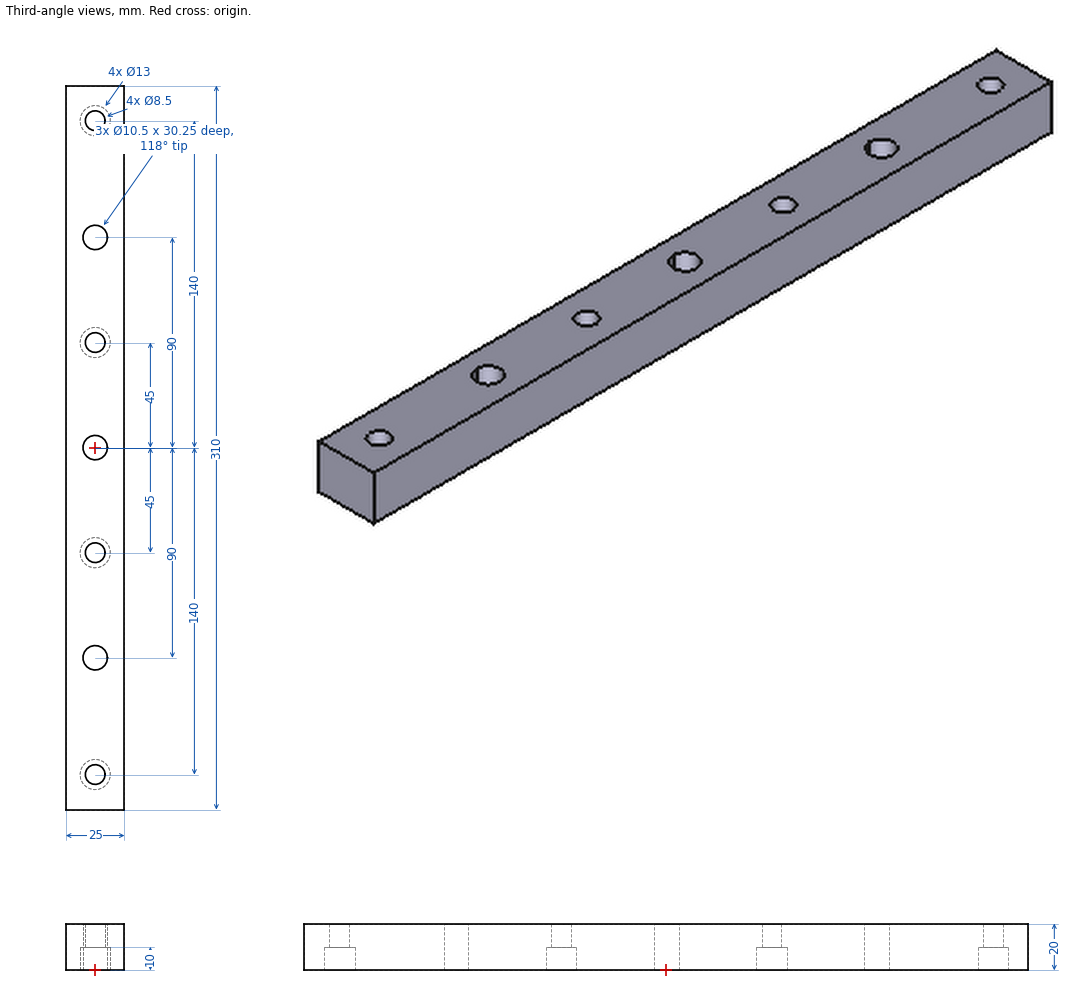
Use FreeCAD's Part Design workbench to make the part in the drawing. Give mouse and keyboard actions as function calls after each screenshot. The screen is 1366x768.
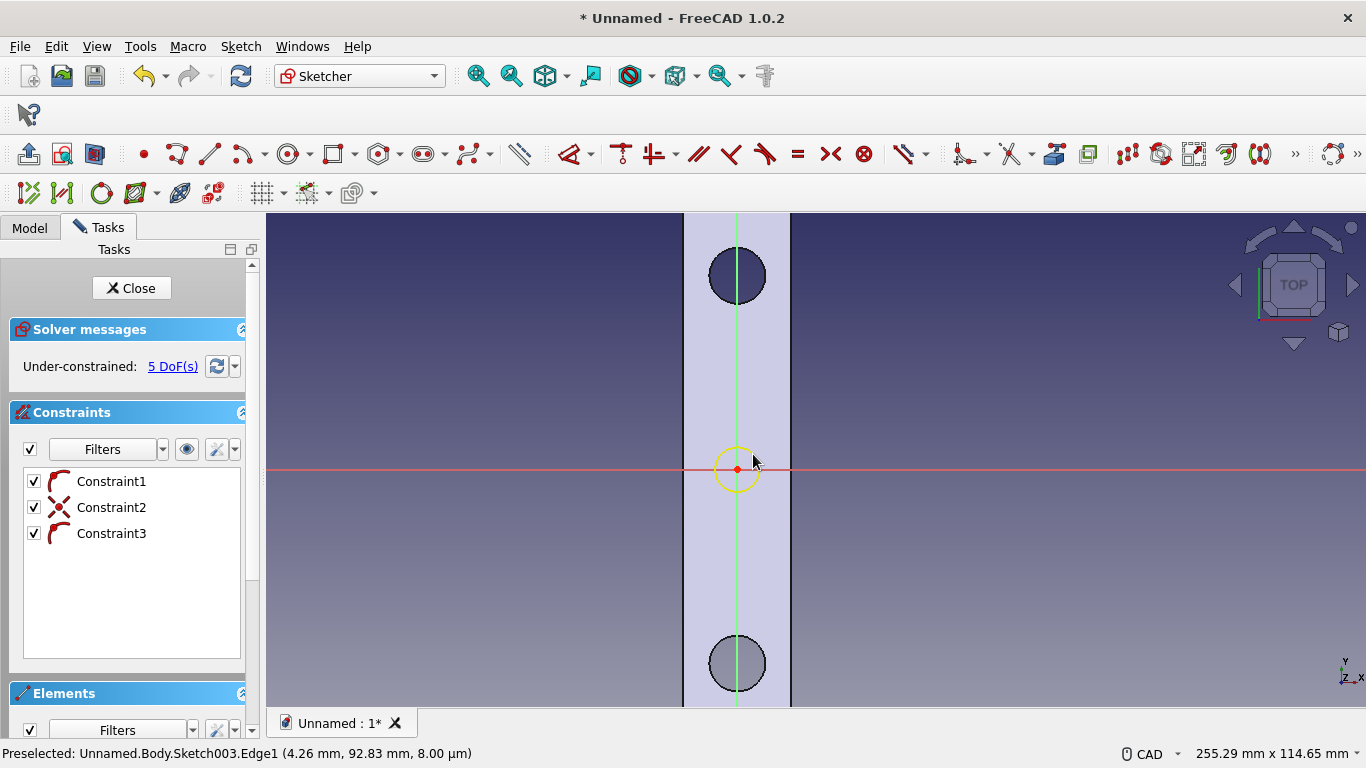
click(753, 454)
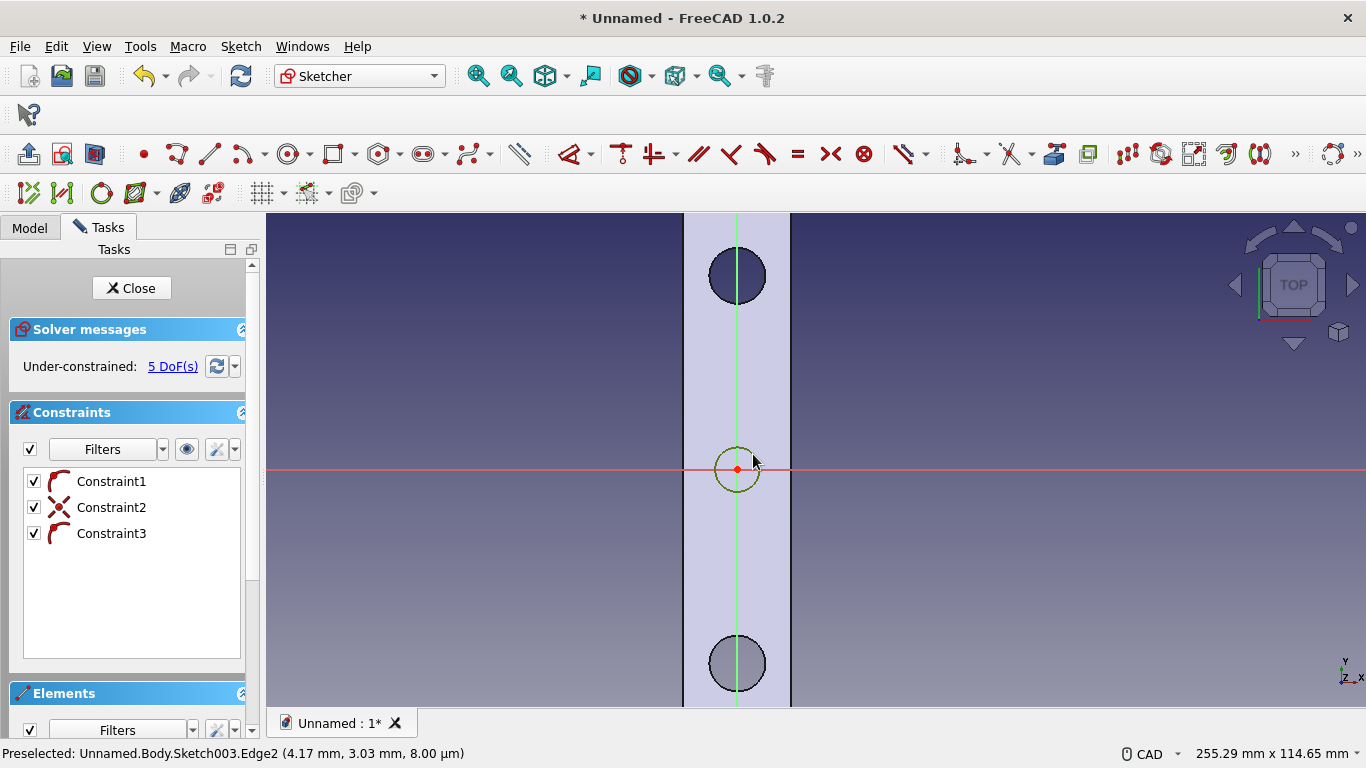
scroll(753, 454, down, 5)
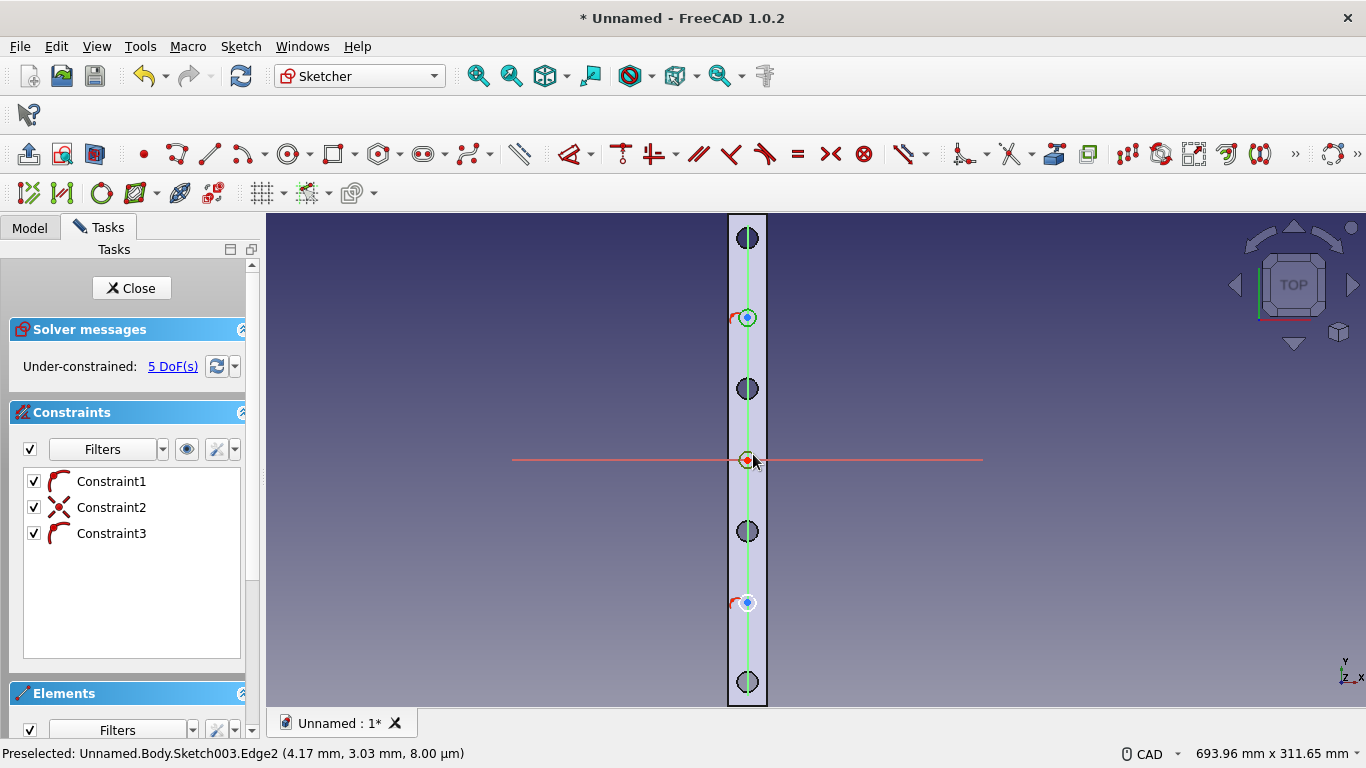
scroll(753, 597, up, 5)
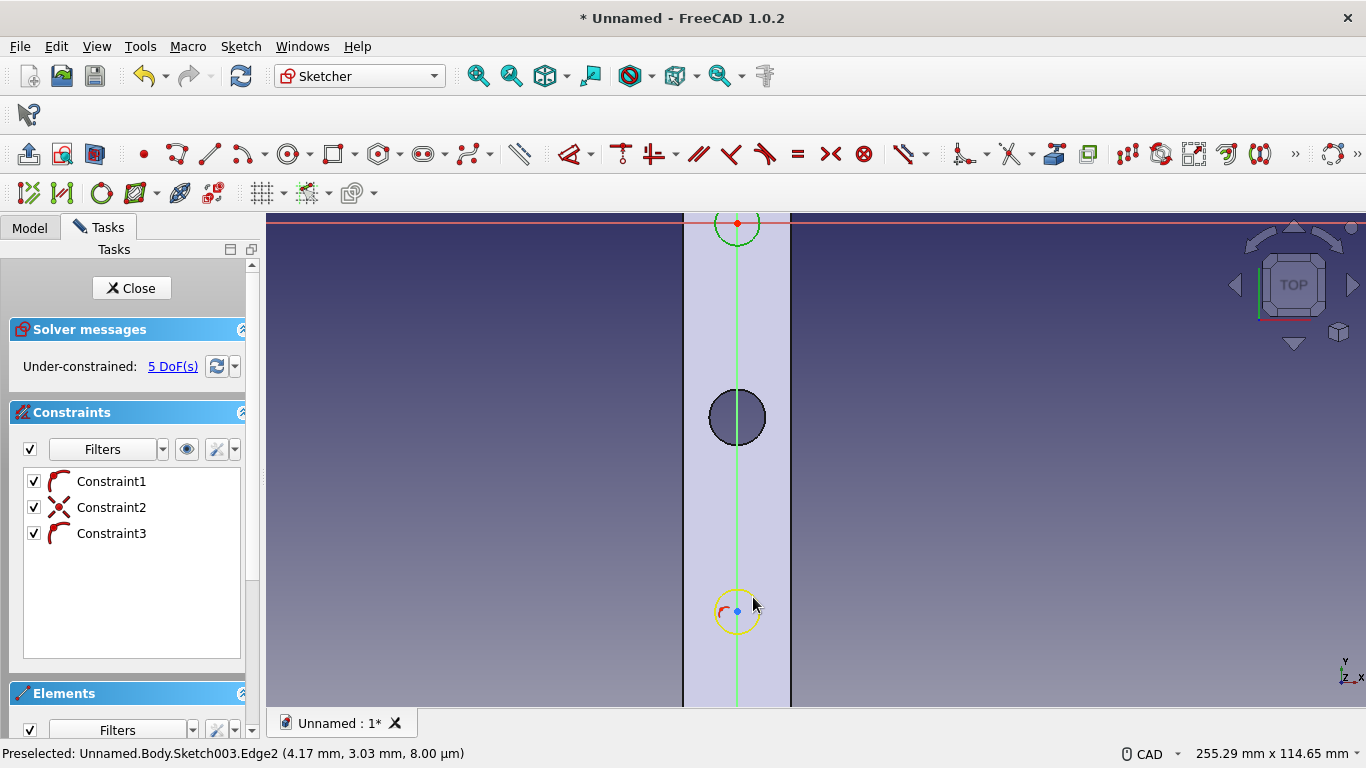
click(753, 596)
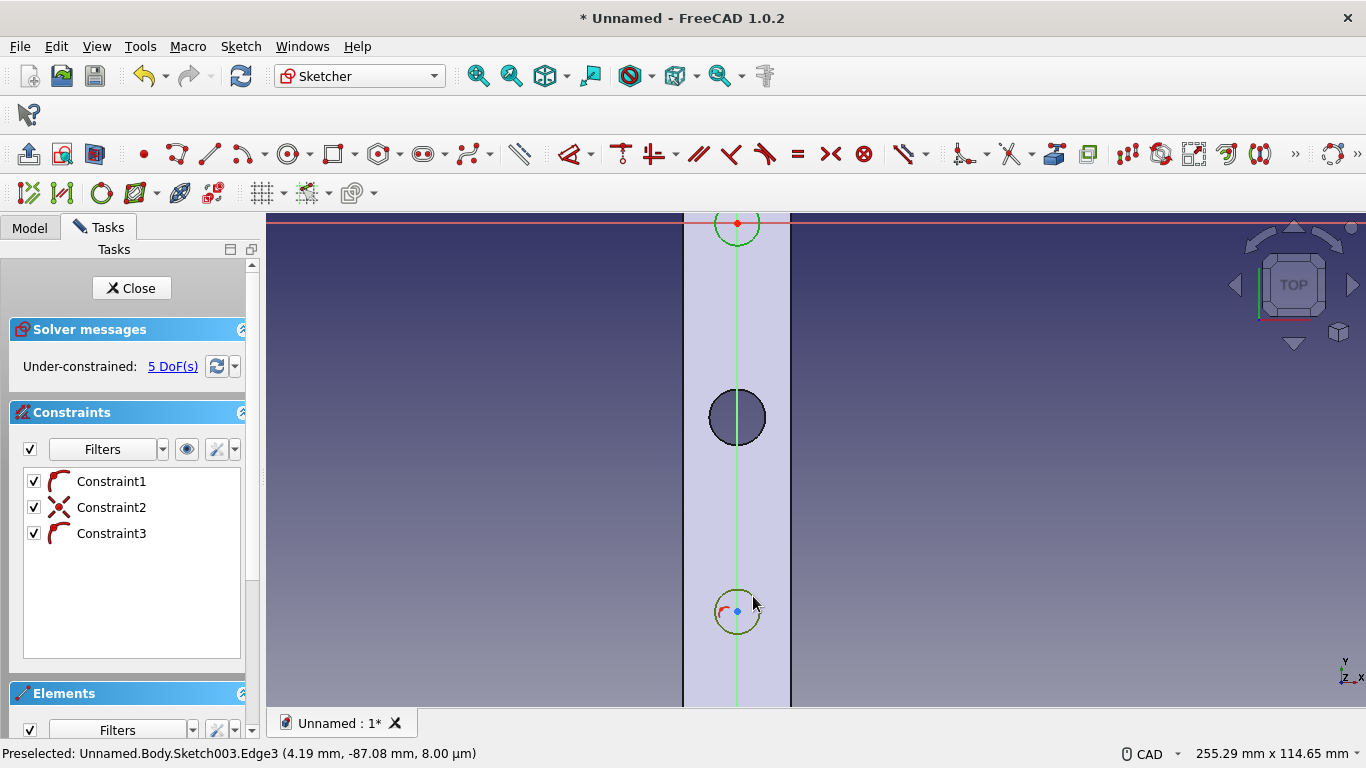
key(e)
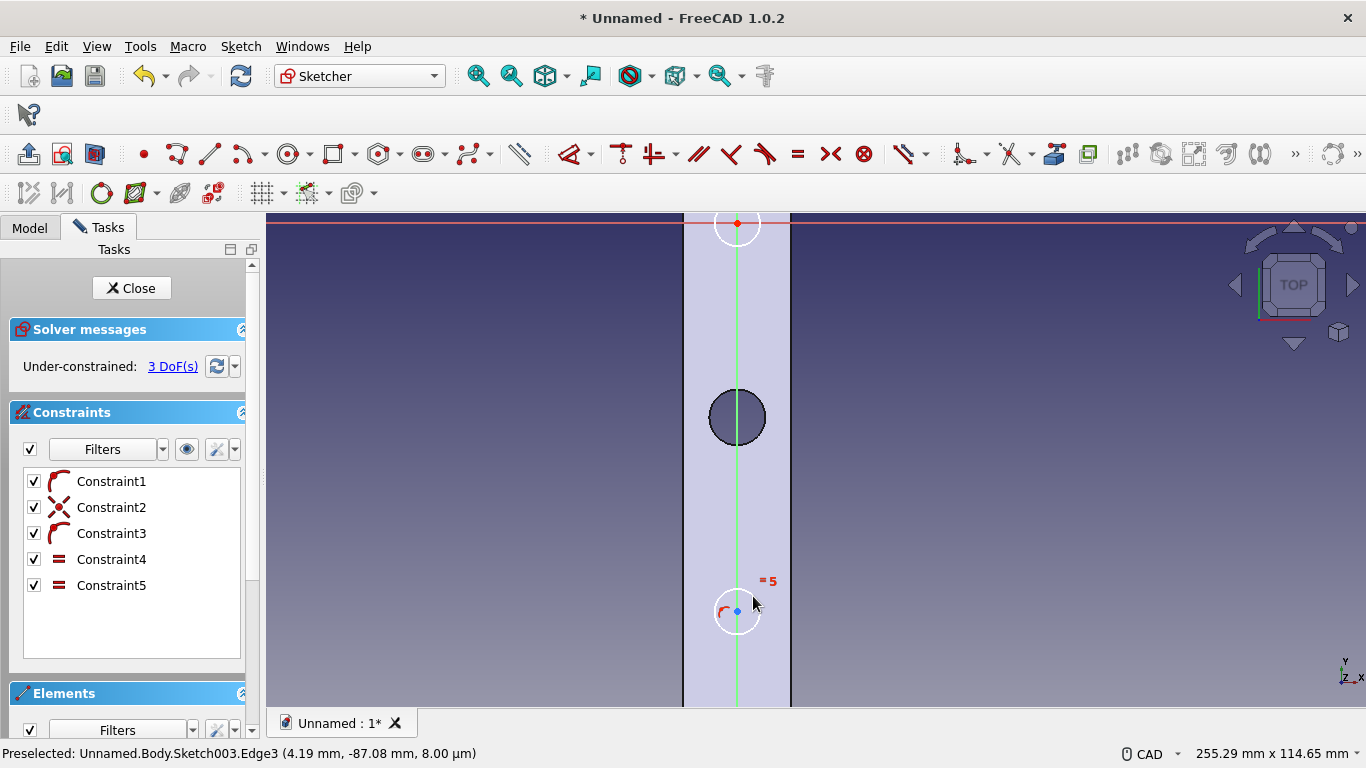
click(568, 154)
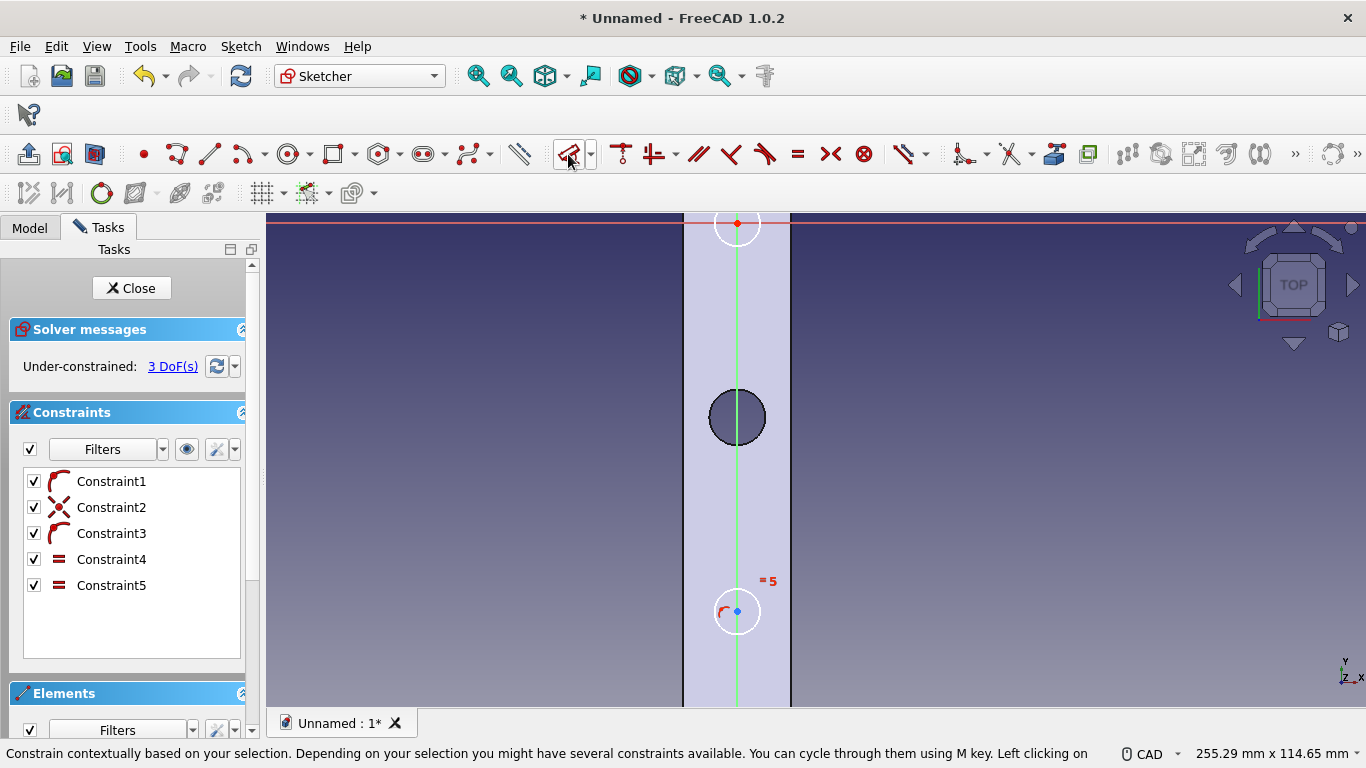
scroll(753, 598, down, 5)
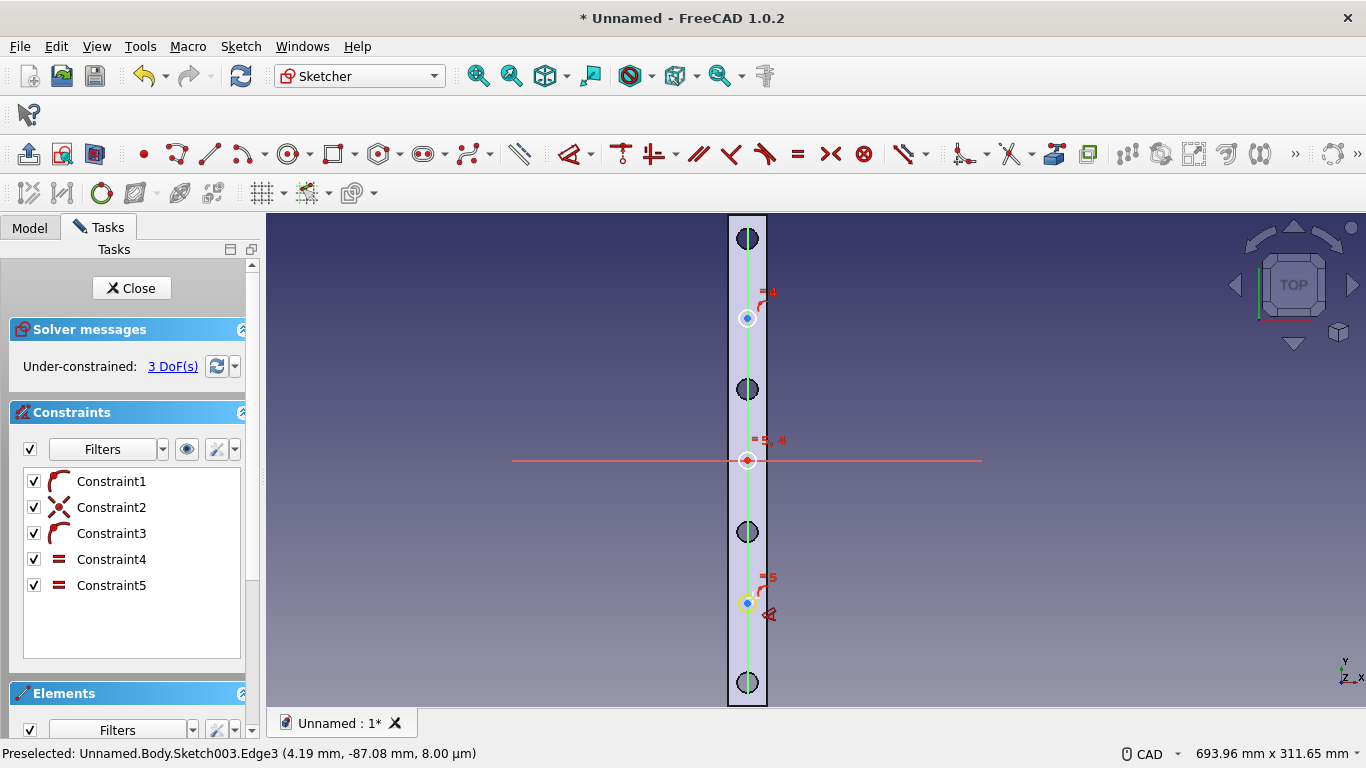
scroll(753, 313, up, 5)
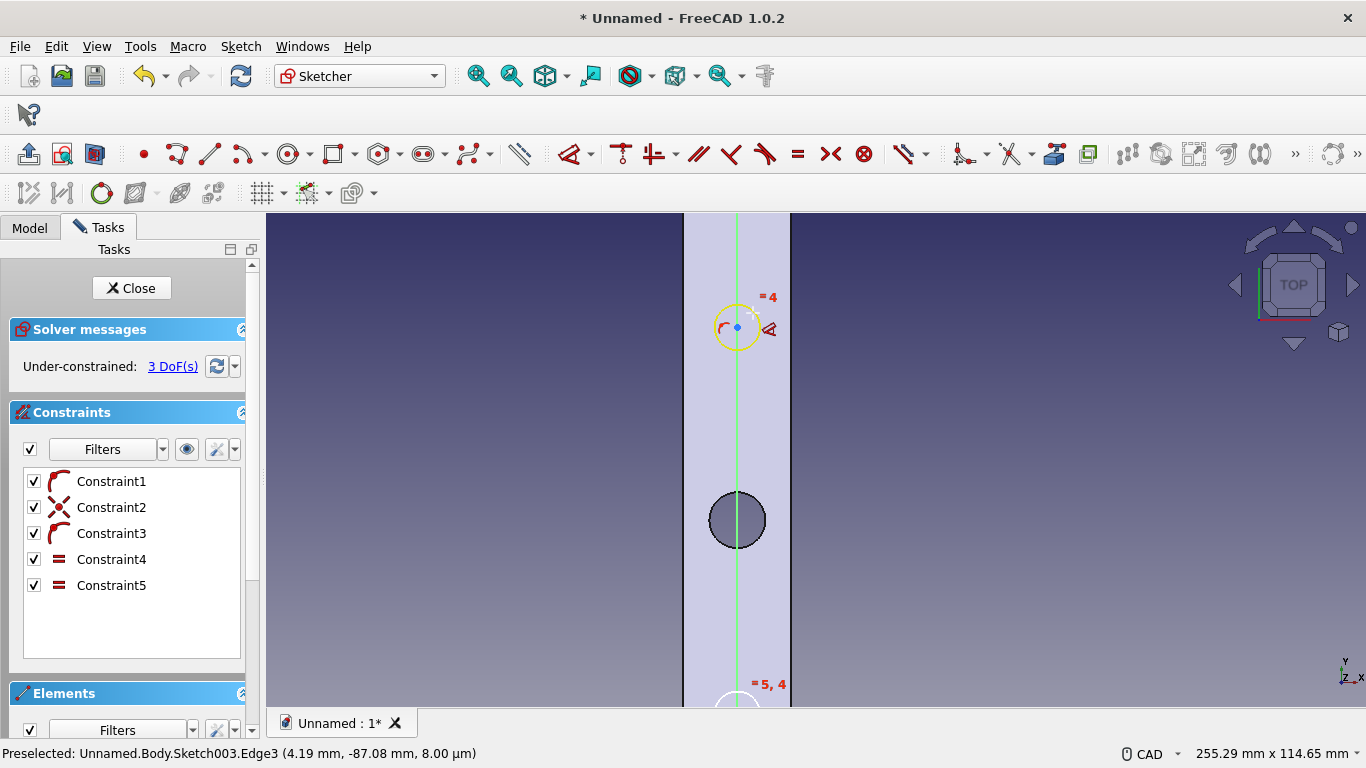
click(753, 311)
click(775, 288)